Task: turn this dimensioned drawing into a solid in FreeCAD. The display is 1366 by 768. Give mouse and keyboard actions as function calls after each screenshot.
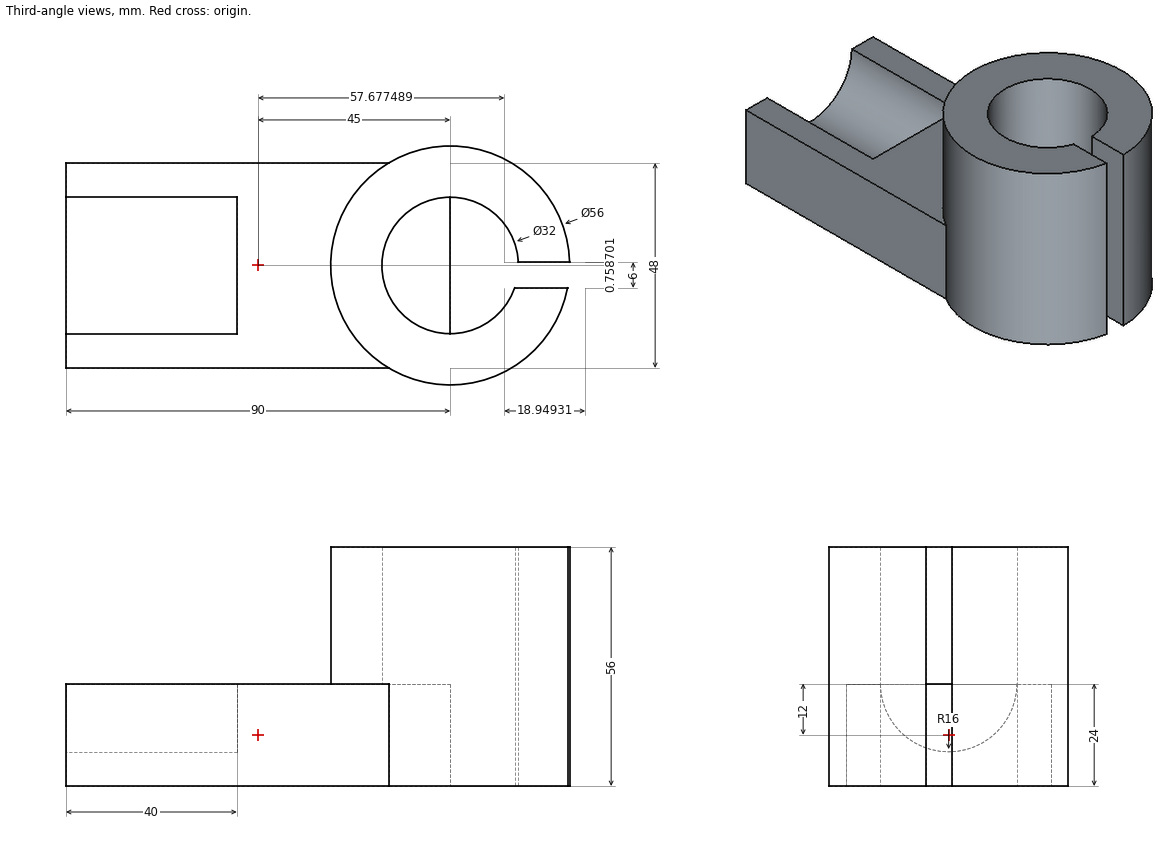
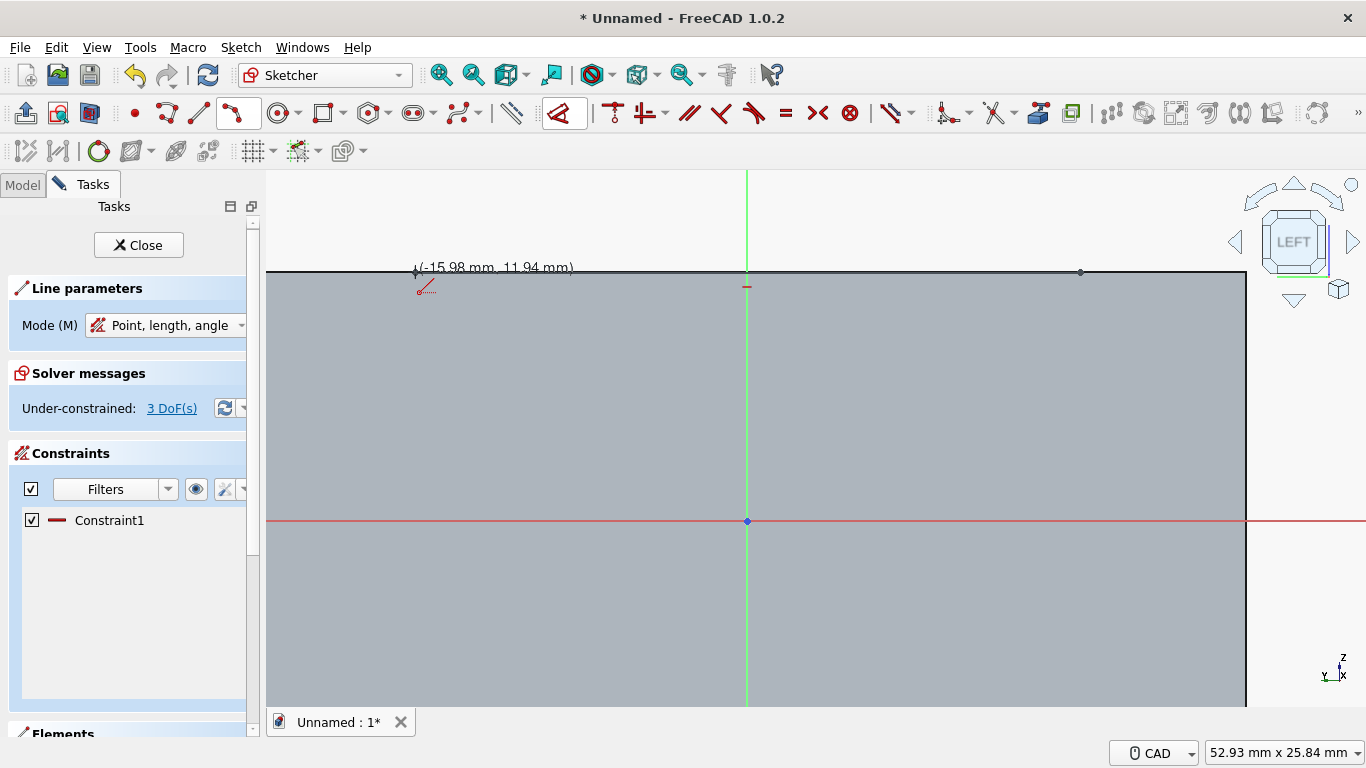
key(g)
key(3)
key(a)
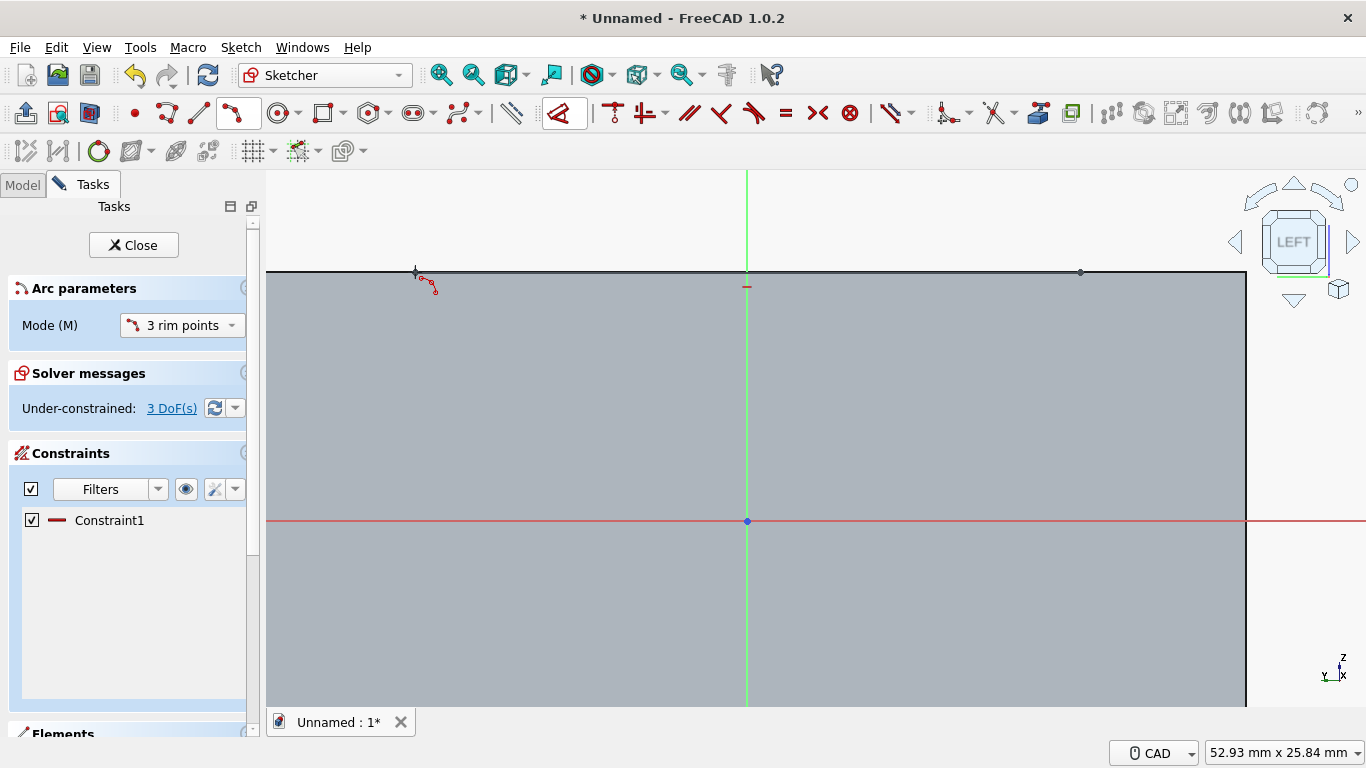
click(415, 273)
click(1080, 273)
click(644, 588)
key(Escape)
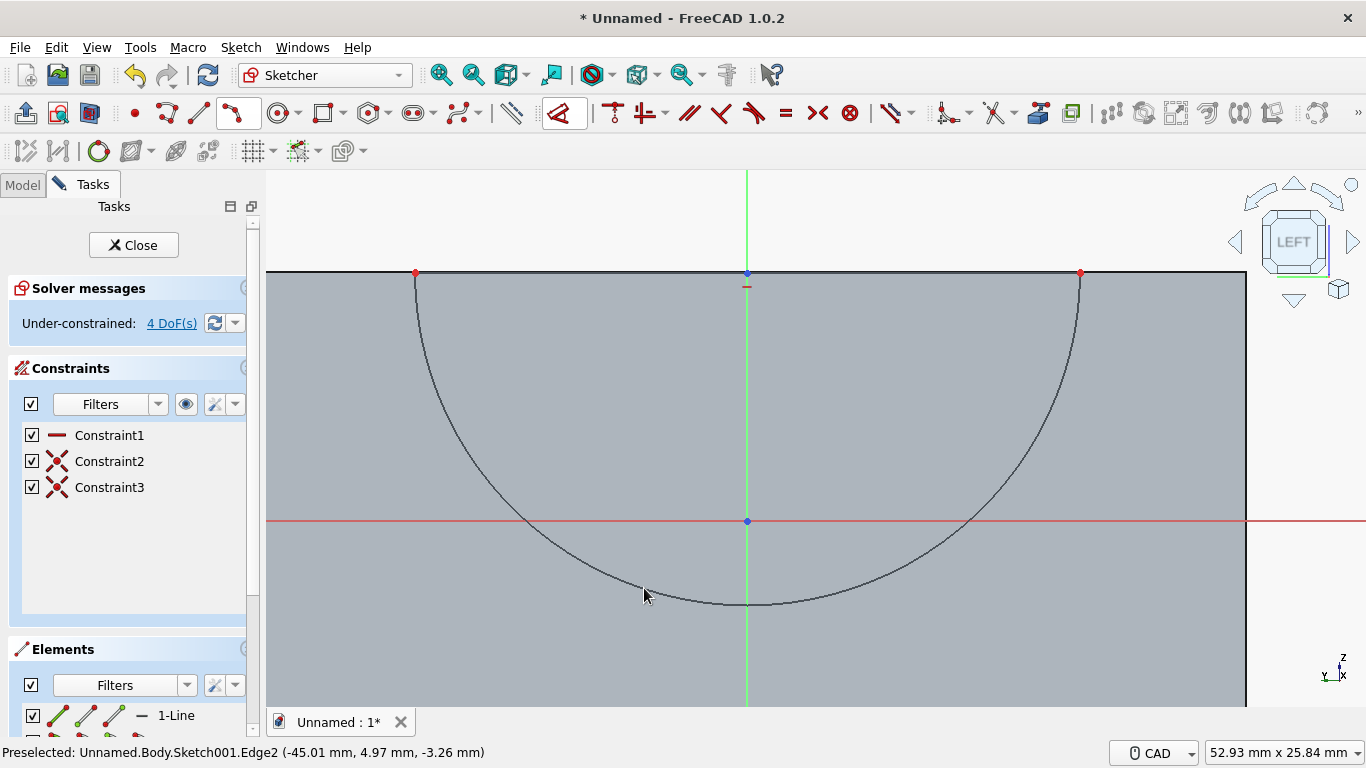
click(748, 273)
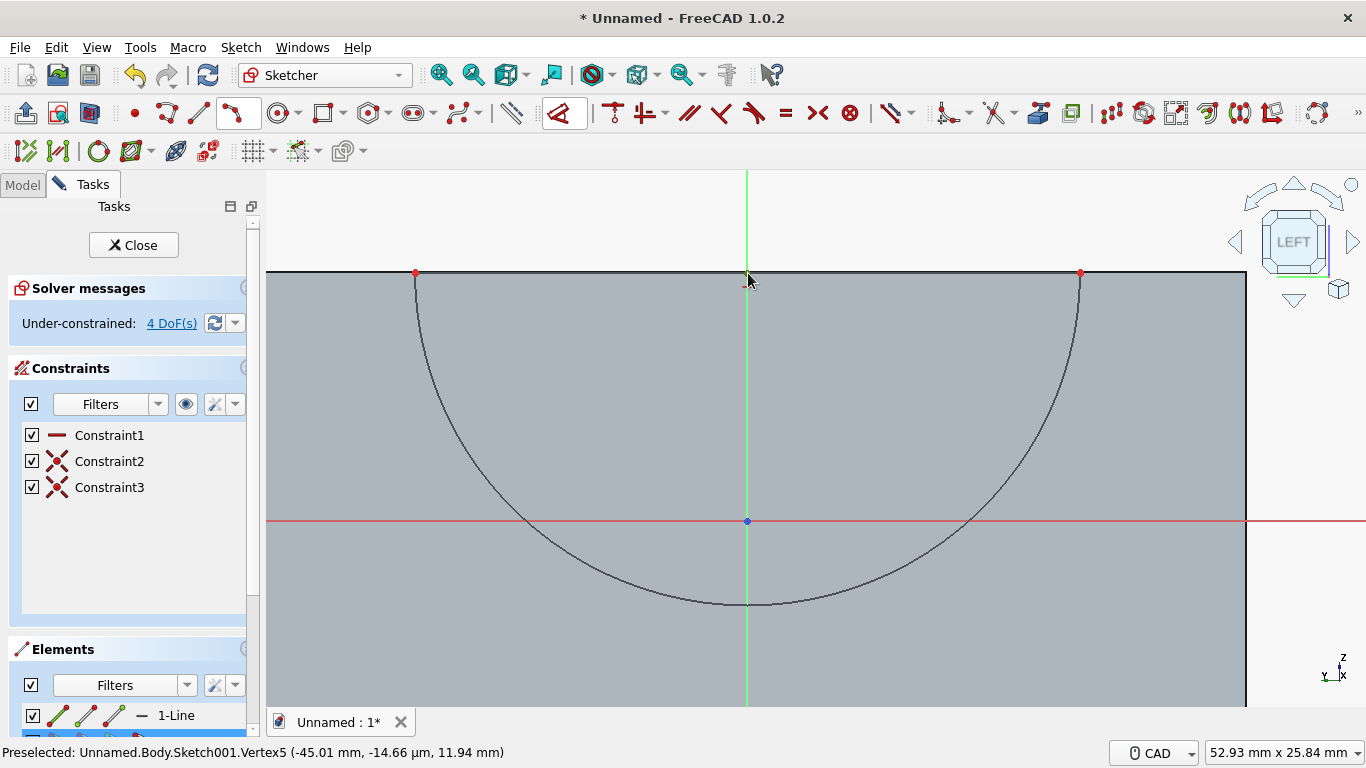
click(747, 645)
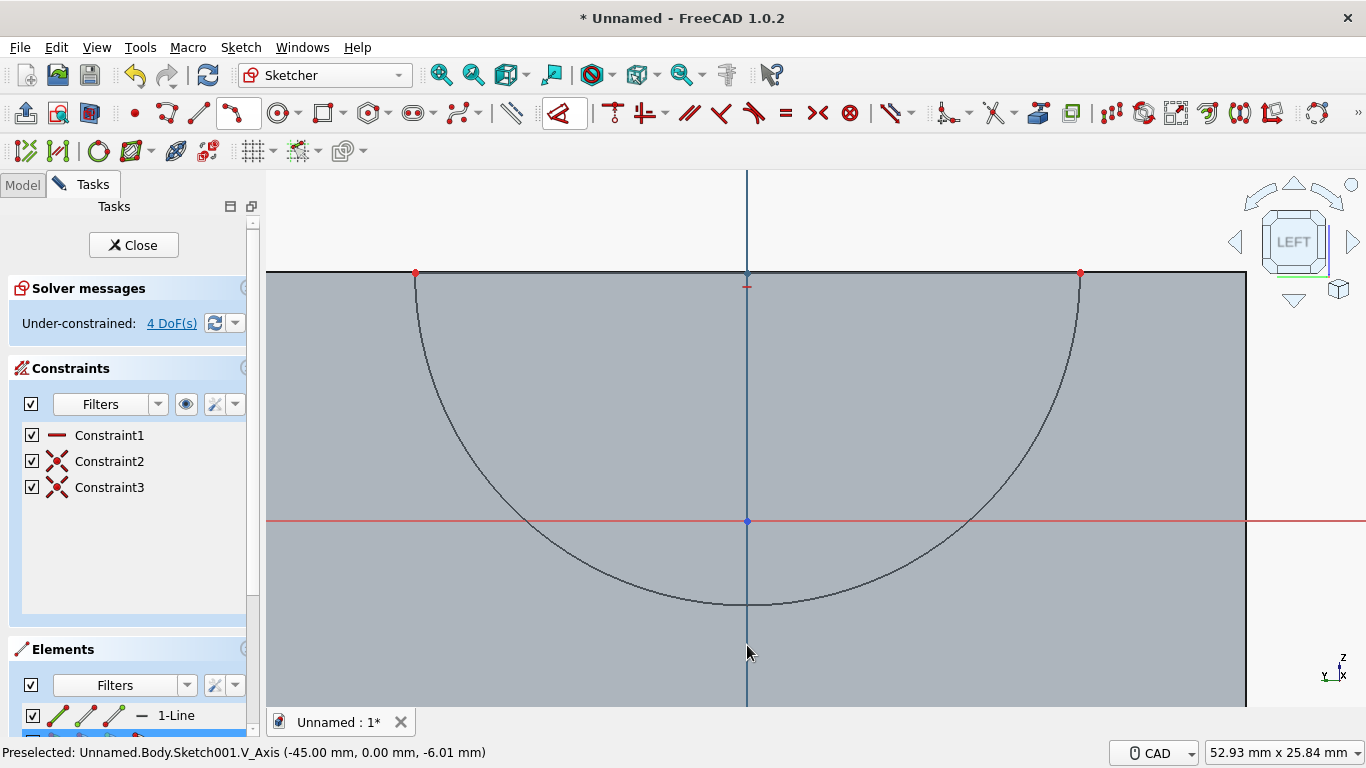
key(c)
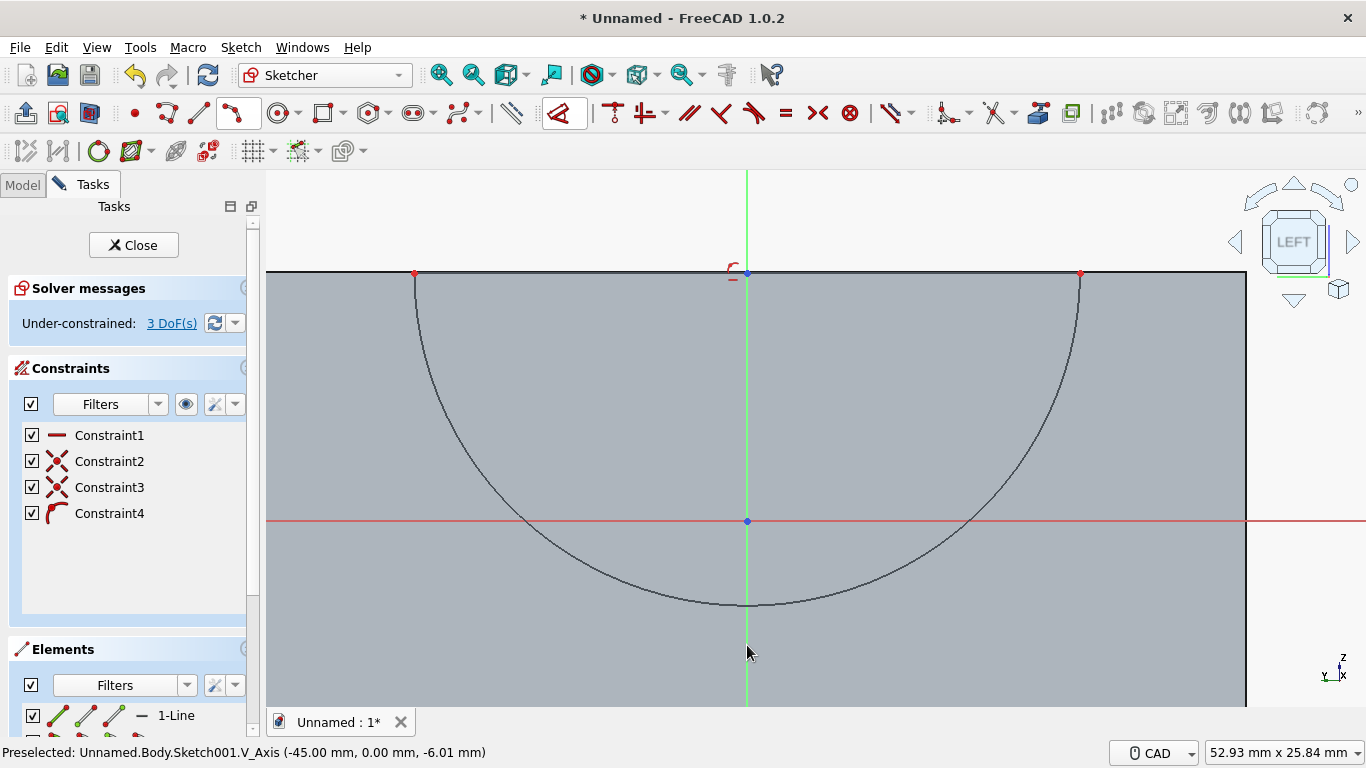
key(d)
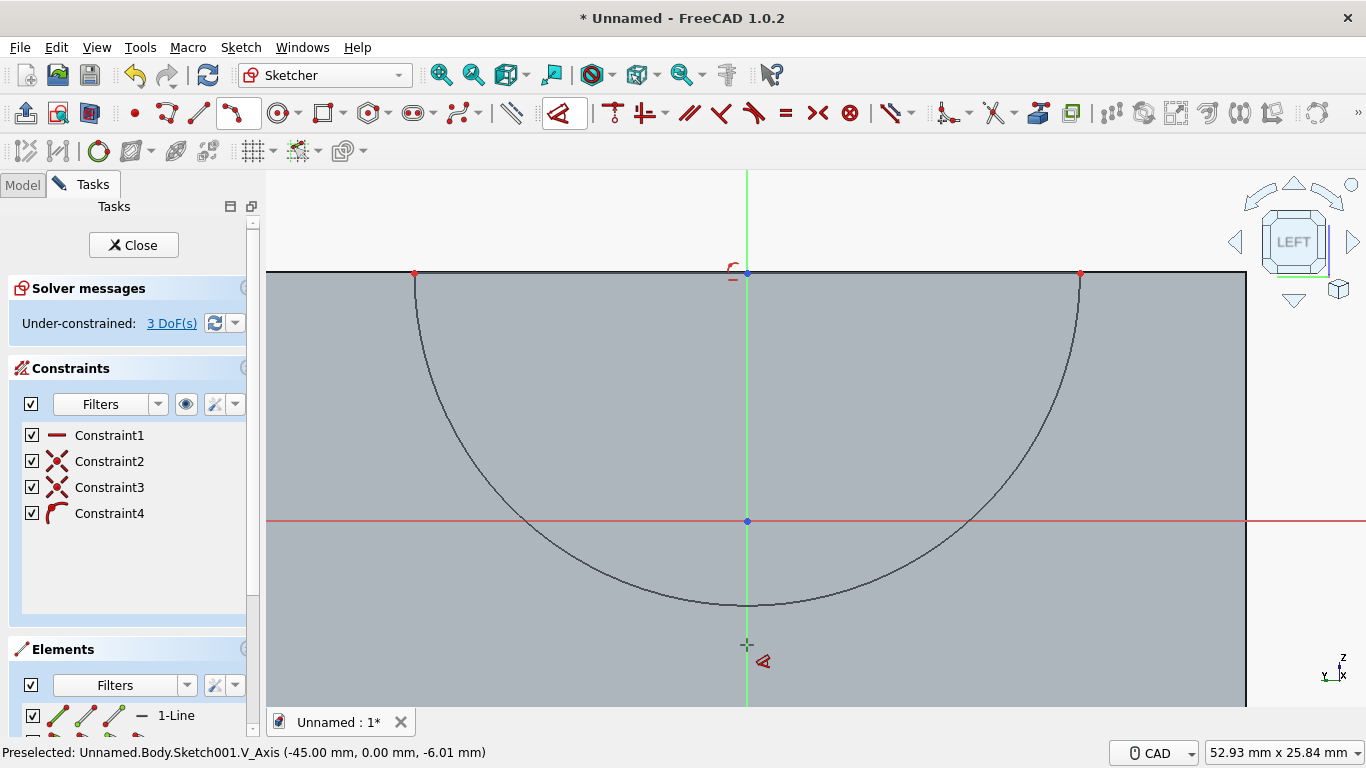
click(552, 542)
click(533, 568)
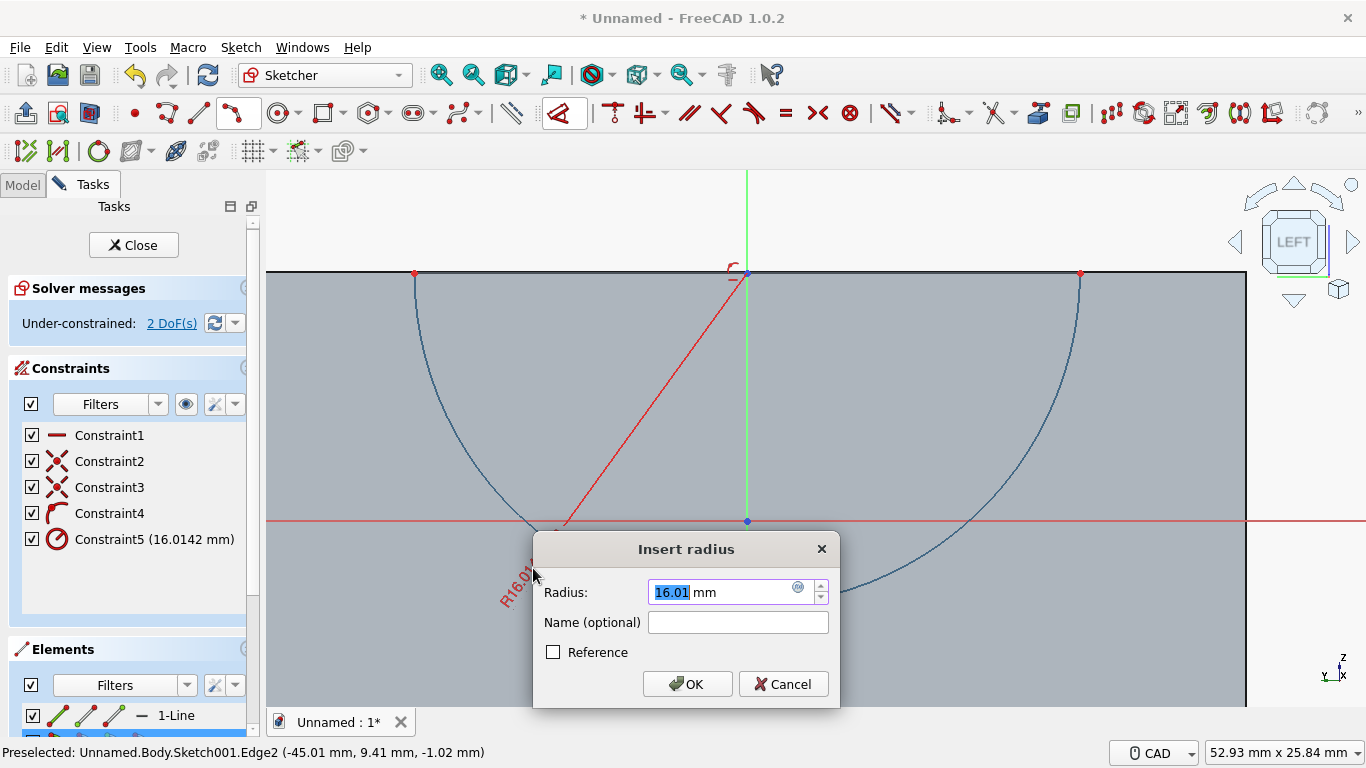
text(16)
key(Return)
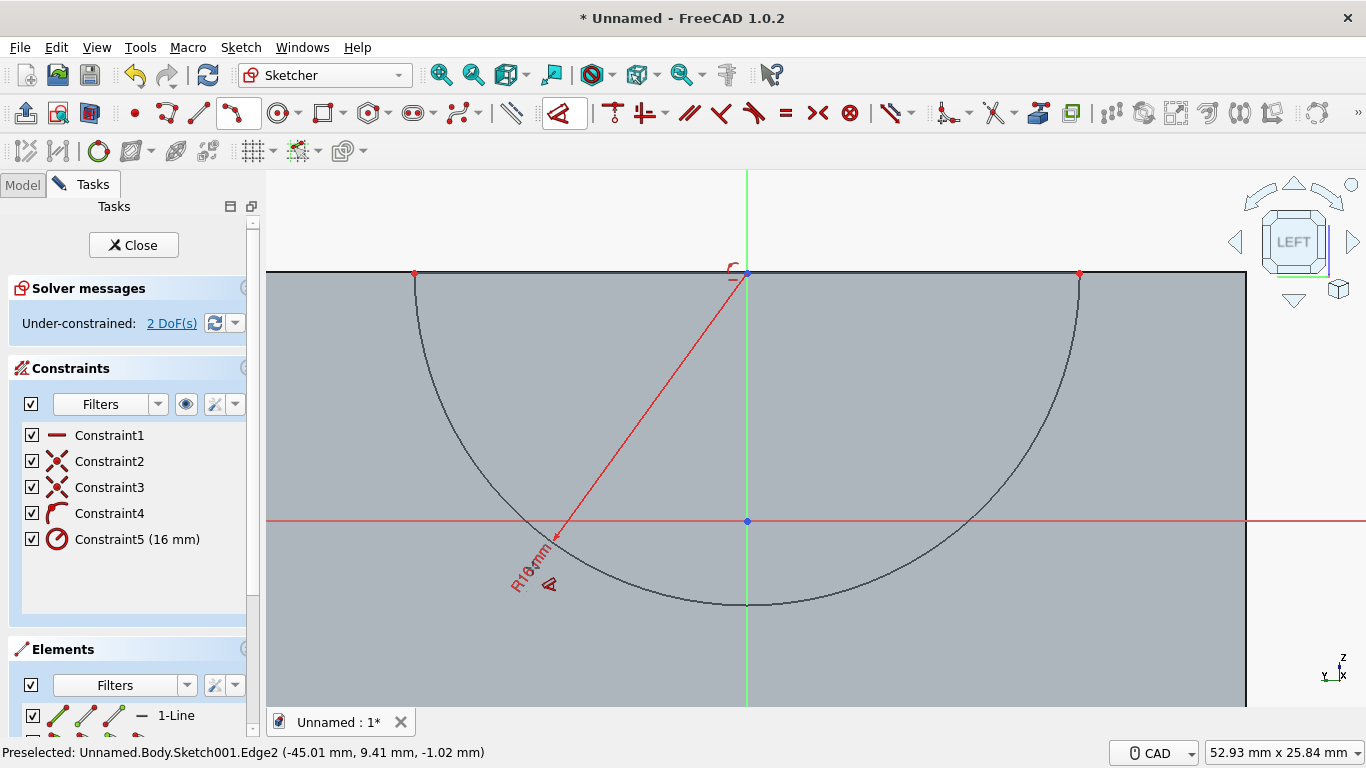
click(1080, 273)
click(1114, 397)